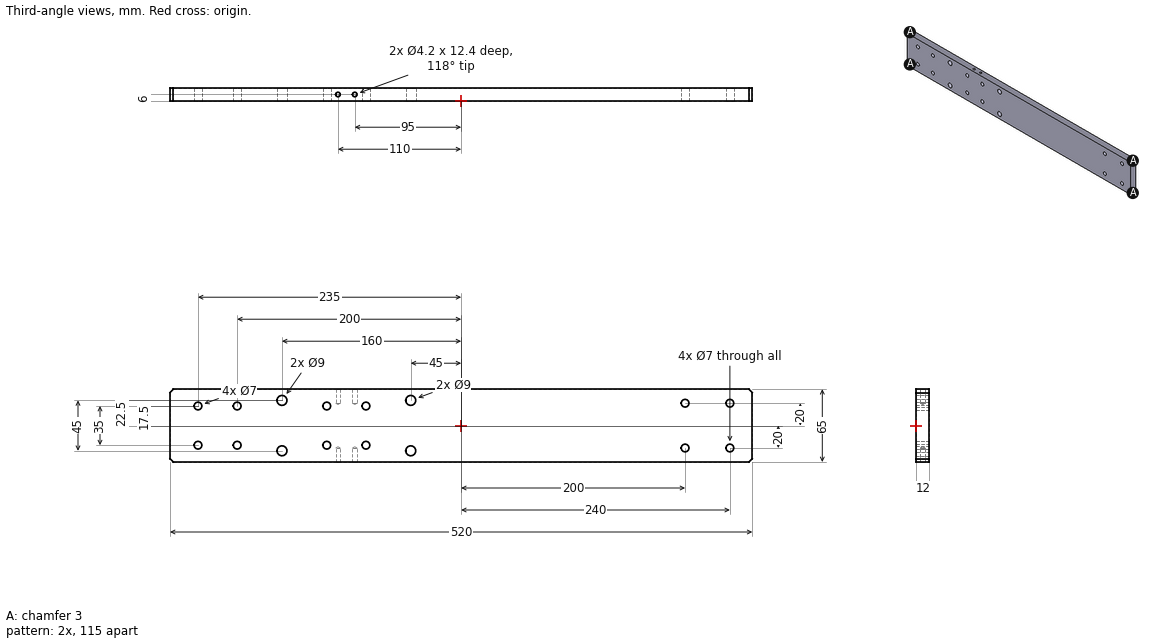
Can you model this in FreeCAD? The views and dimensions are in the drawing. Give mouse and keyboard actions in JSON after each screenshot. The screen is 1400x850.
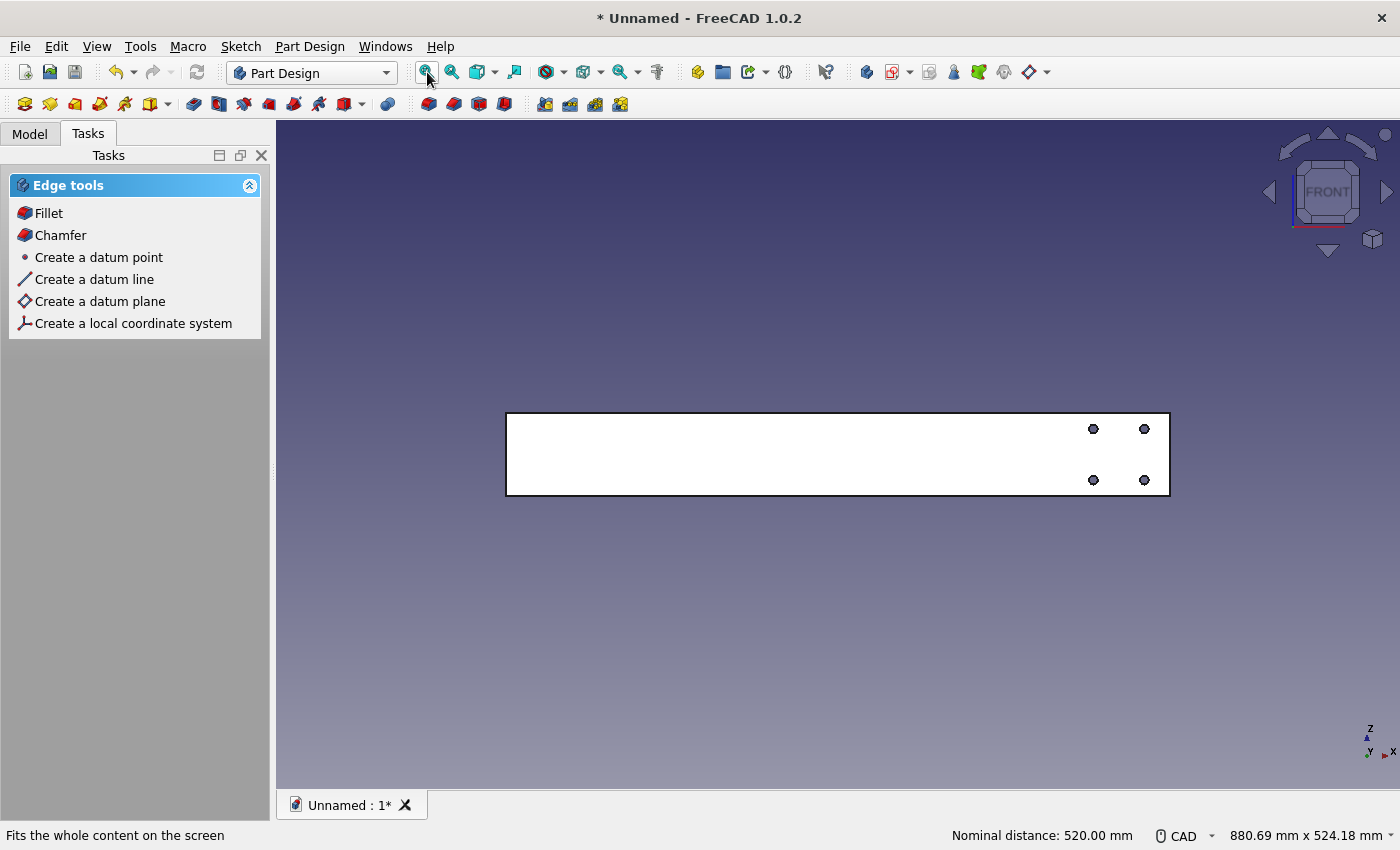
{"action": "scroll", "coordinate": [506, 495], "scroll_direction": "up", "scroll_amount": 5}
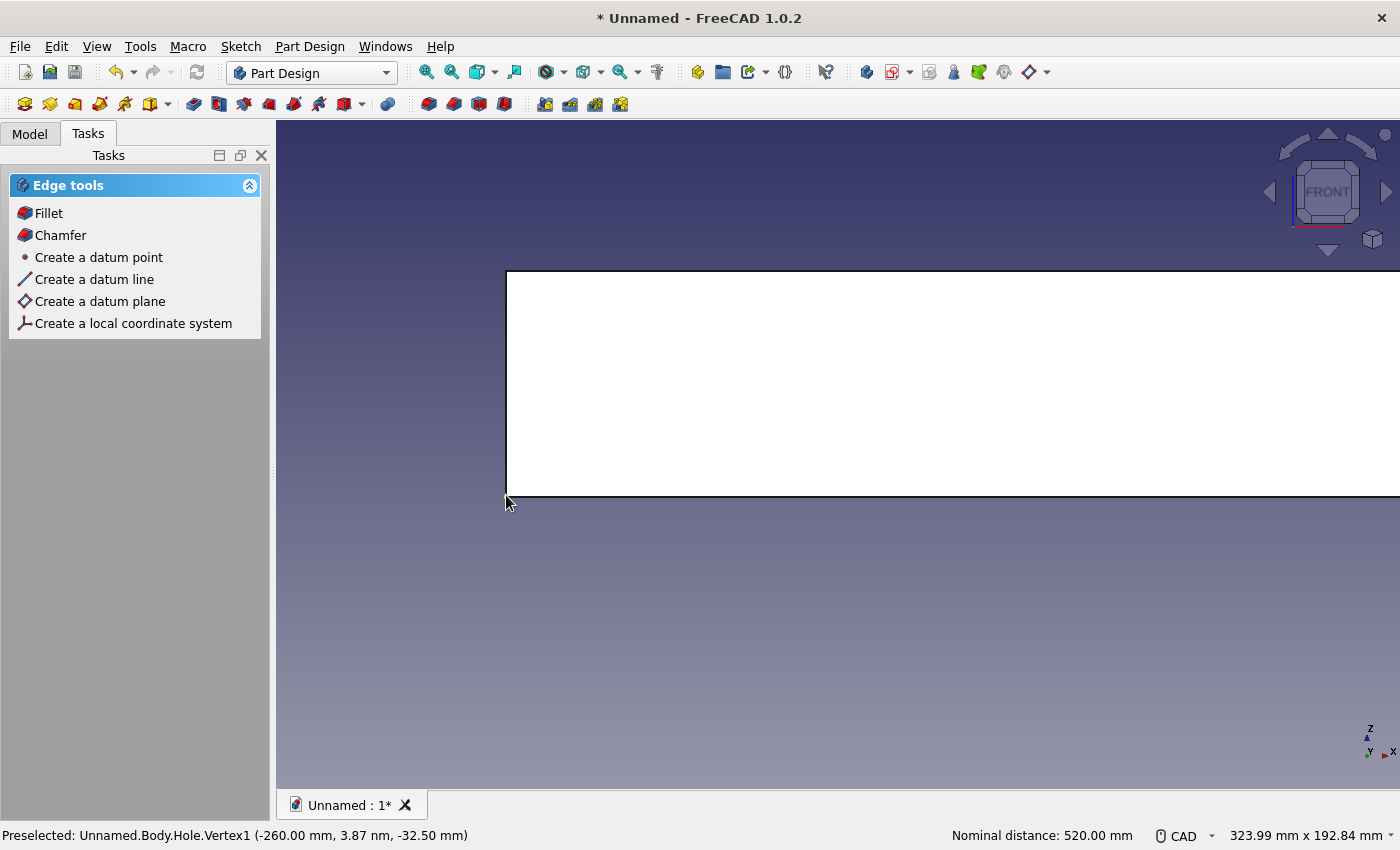
{"action": "key", "text": "v f"}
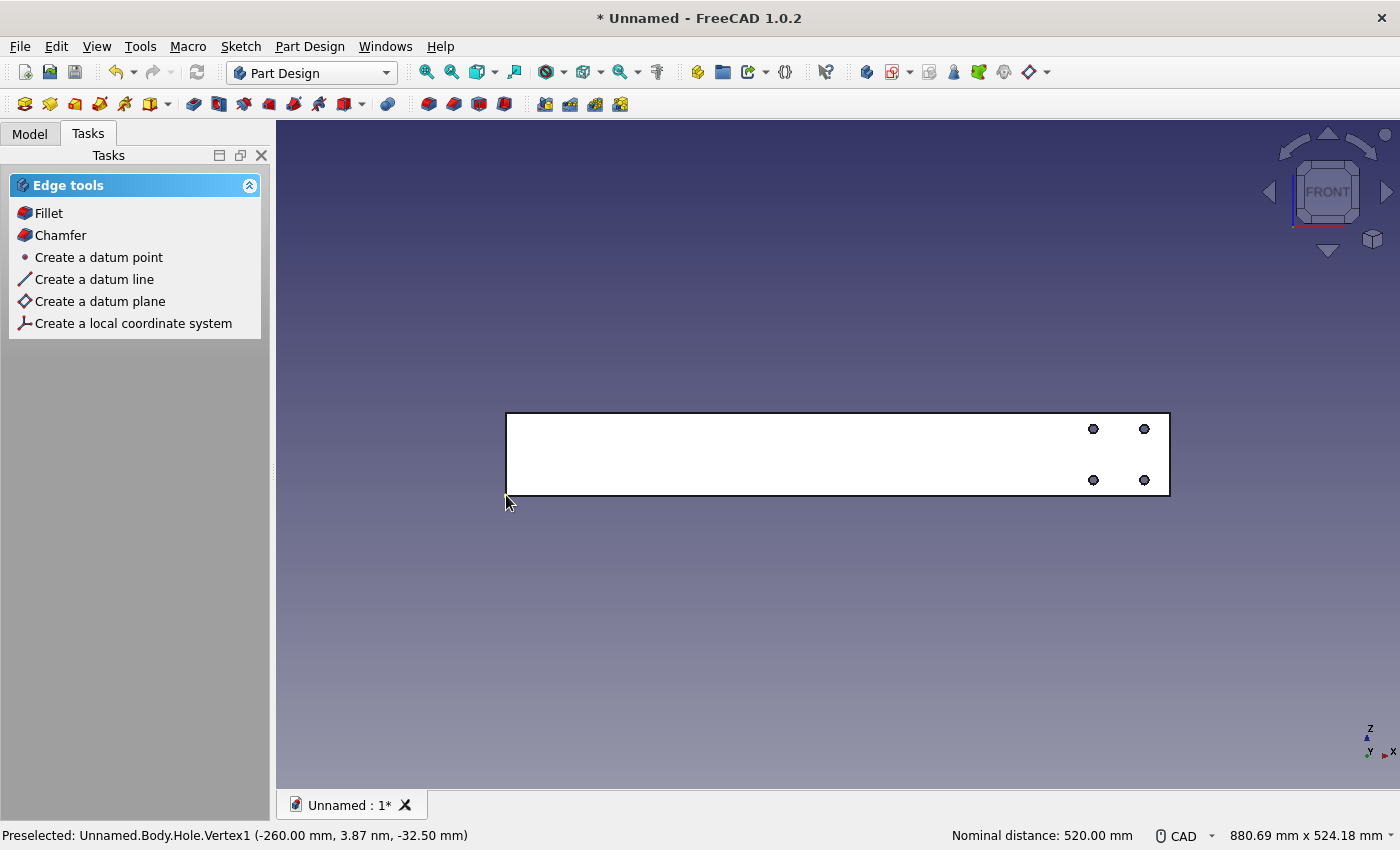
{"action": "key", "text": "3"}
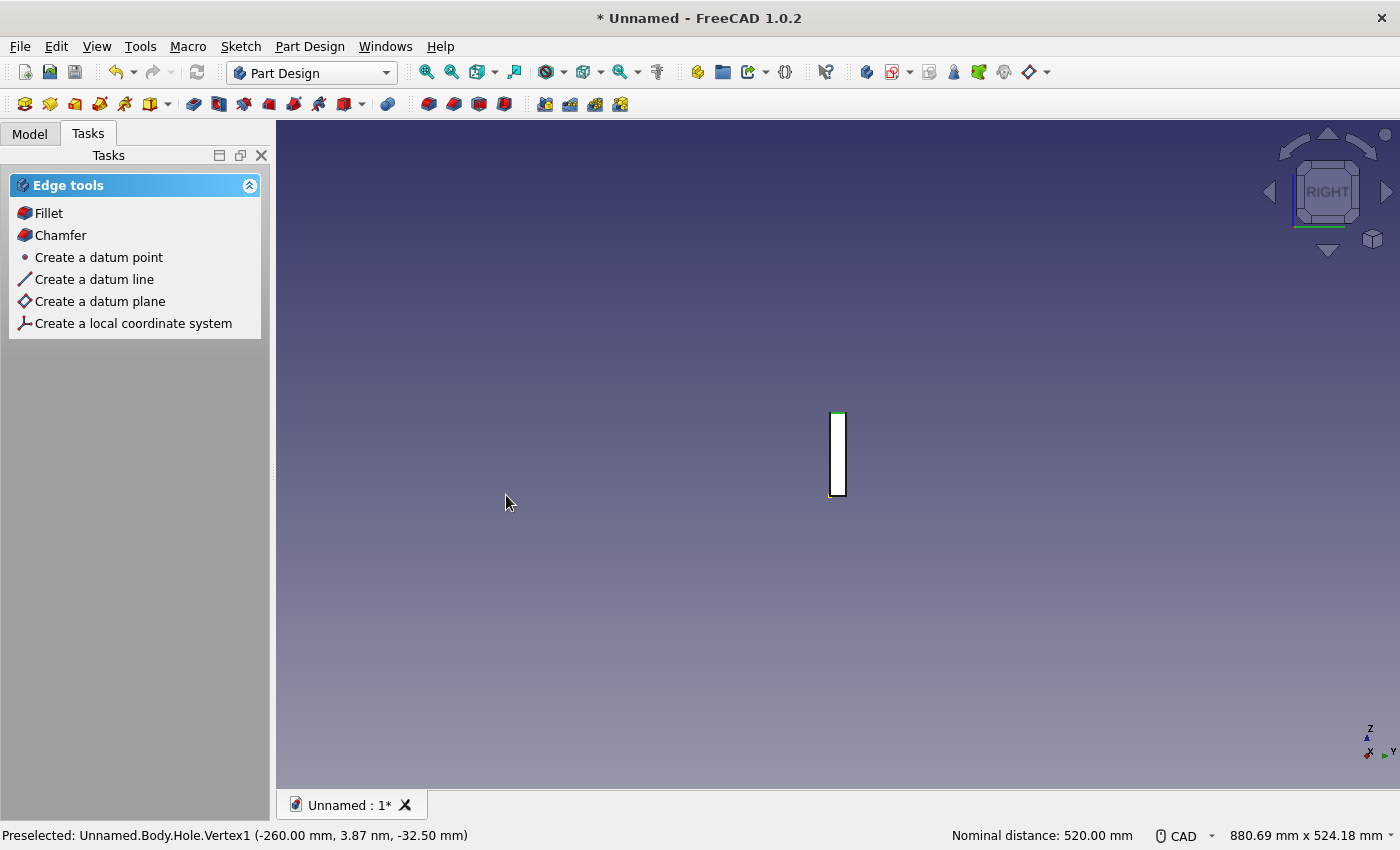
{"action": "left_click", "coordinate": [427, 72]}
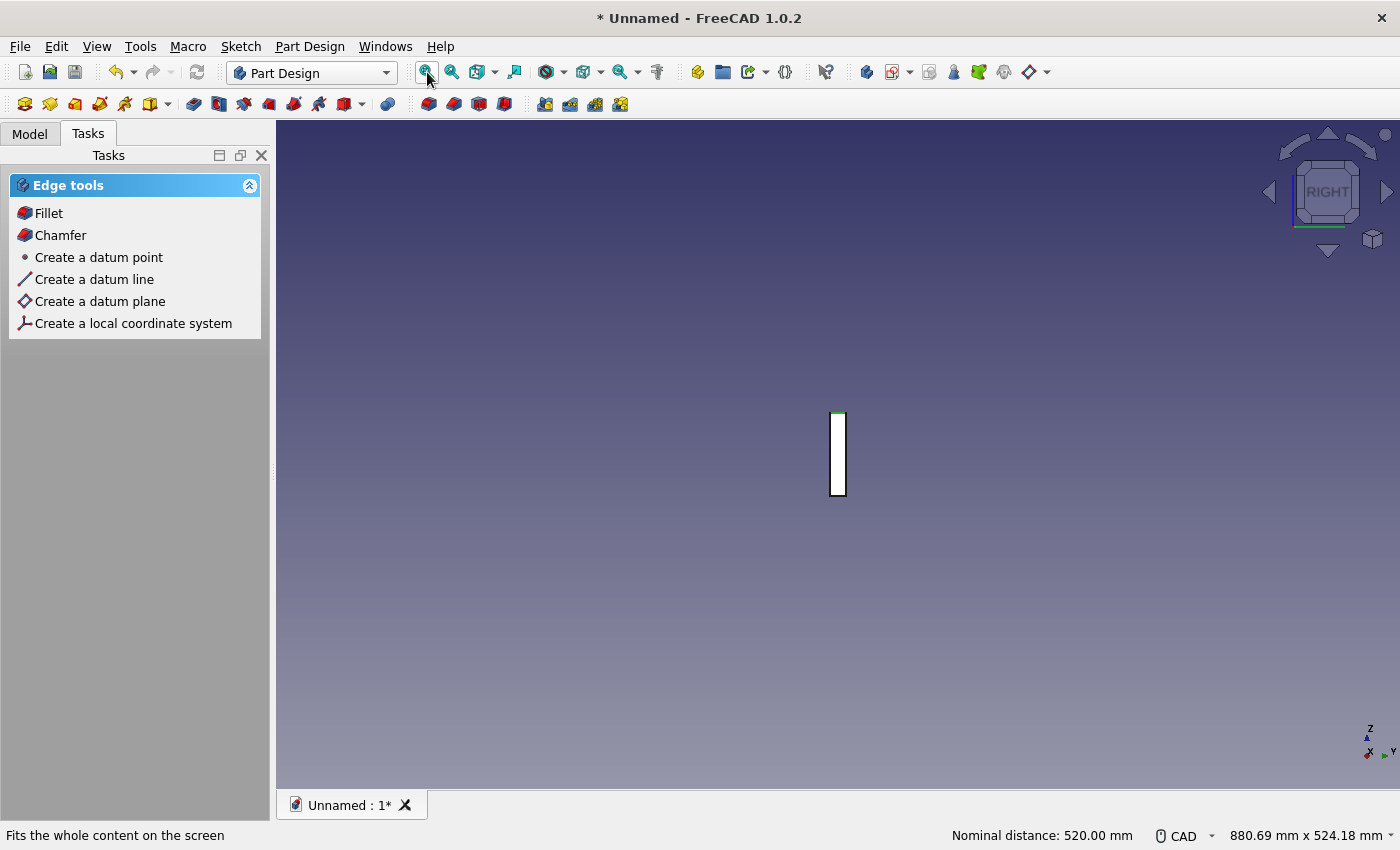
{"action": "left_click", "coordinate": [838, 495], "text": "ctrl"}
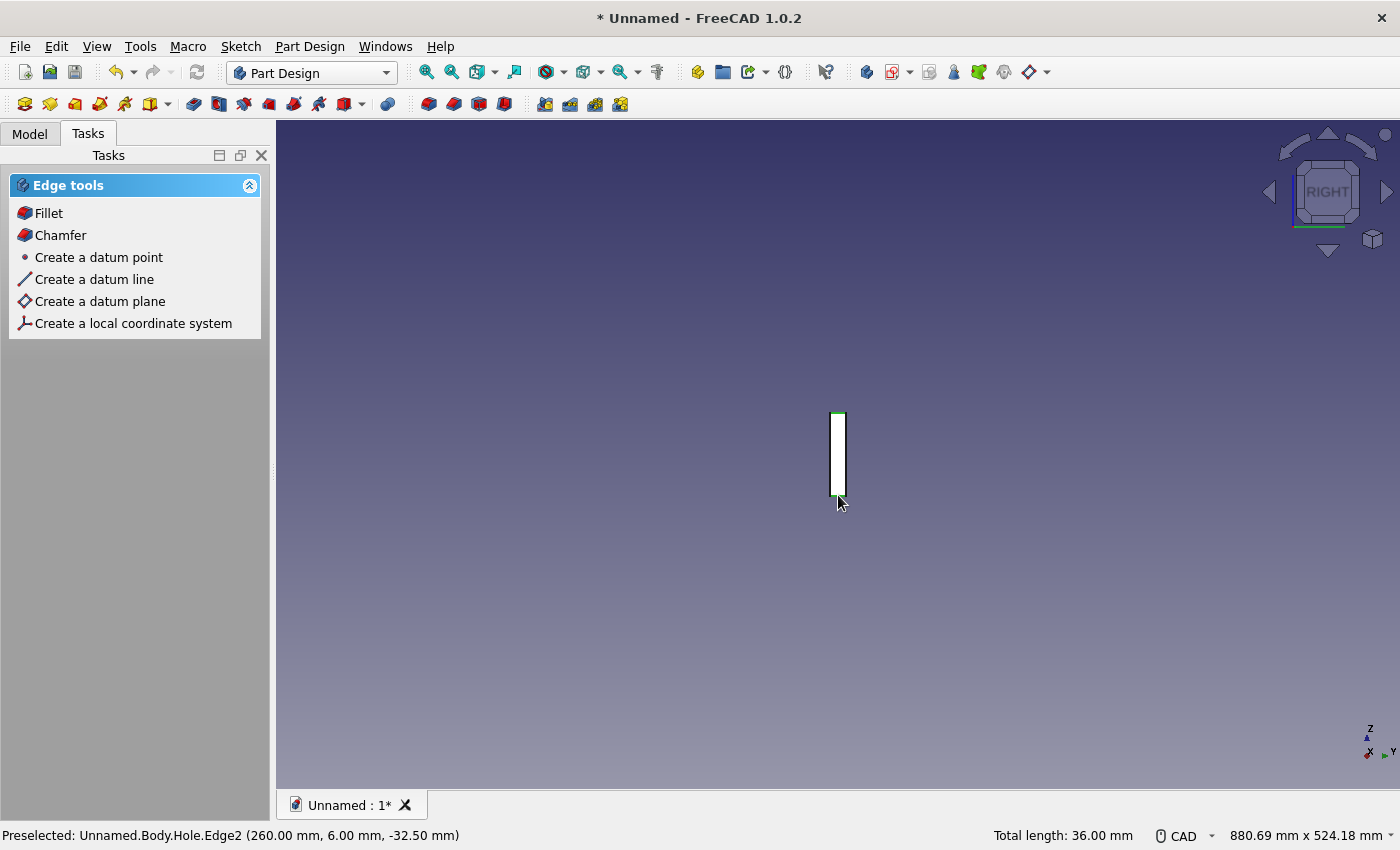
{"action": "scroll", "coordinate": [838, 495], "scroll_direction": "up", "scroll_amount": 5}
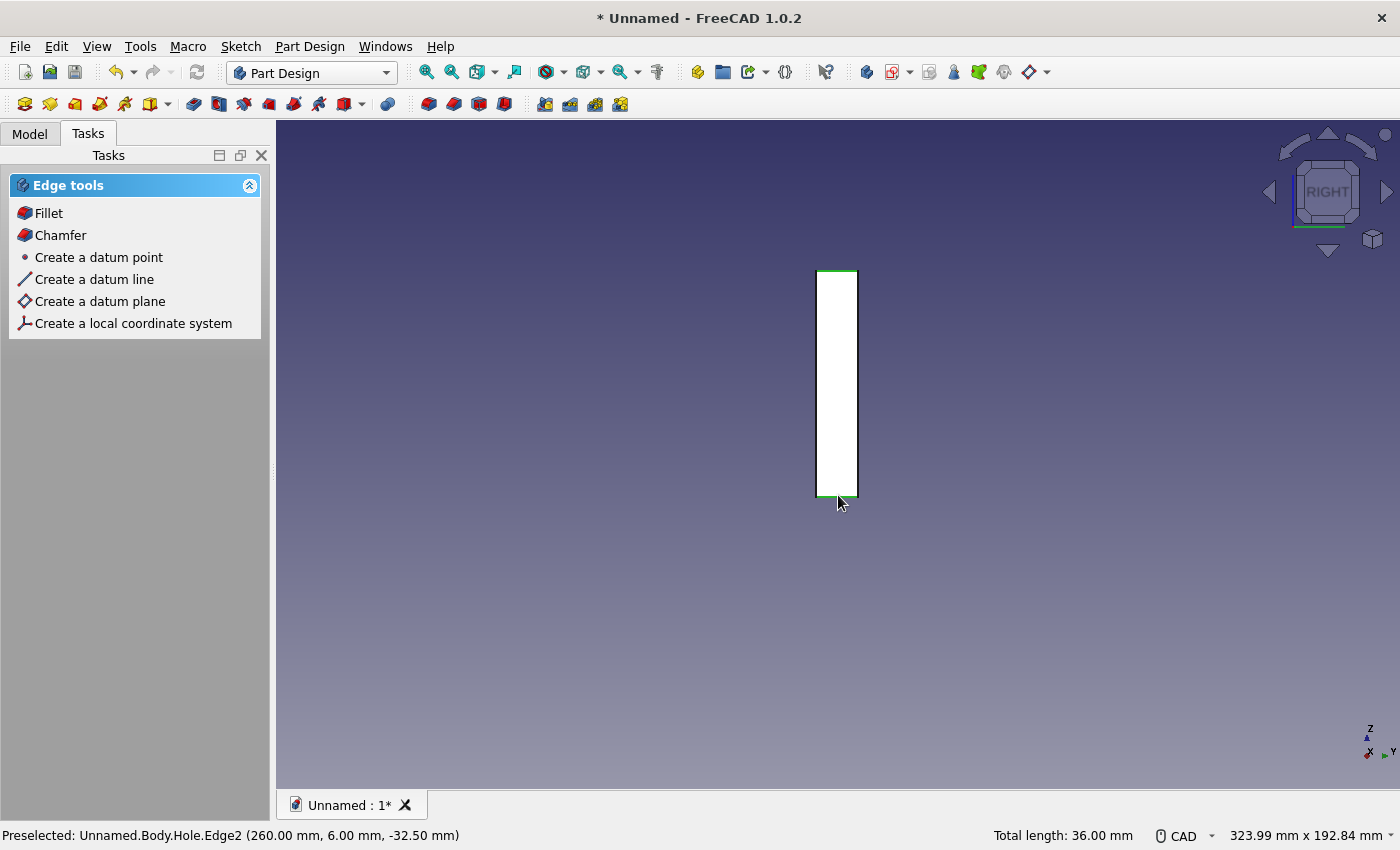
{"action": "left_click", "coordinate": [427, 72]}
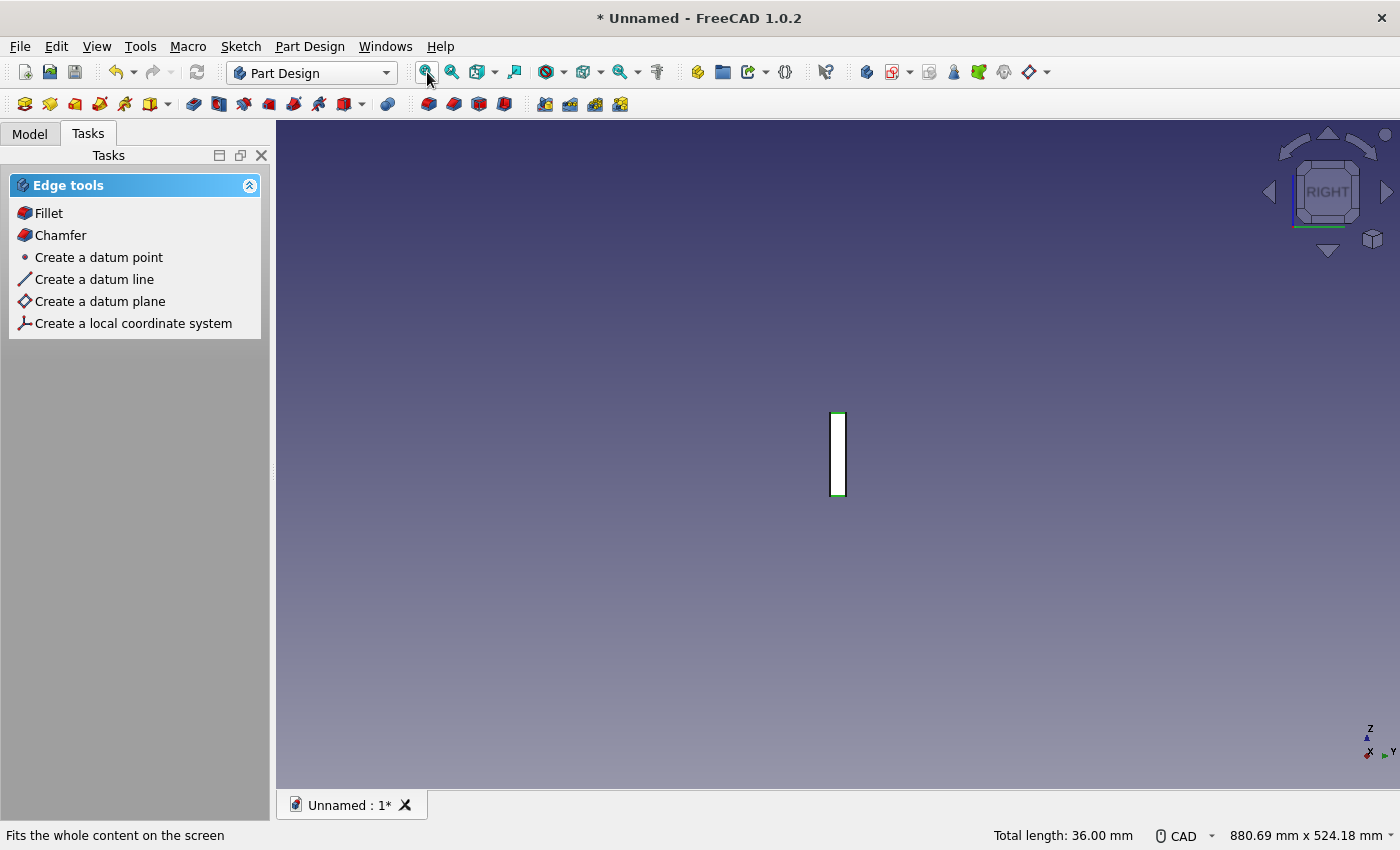
{"action": "key", "text": "5"}